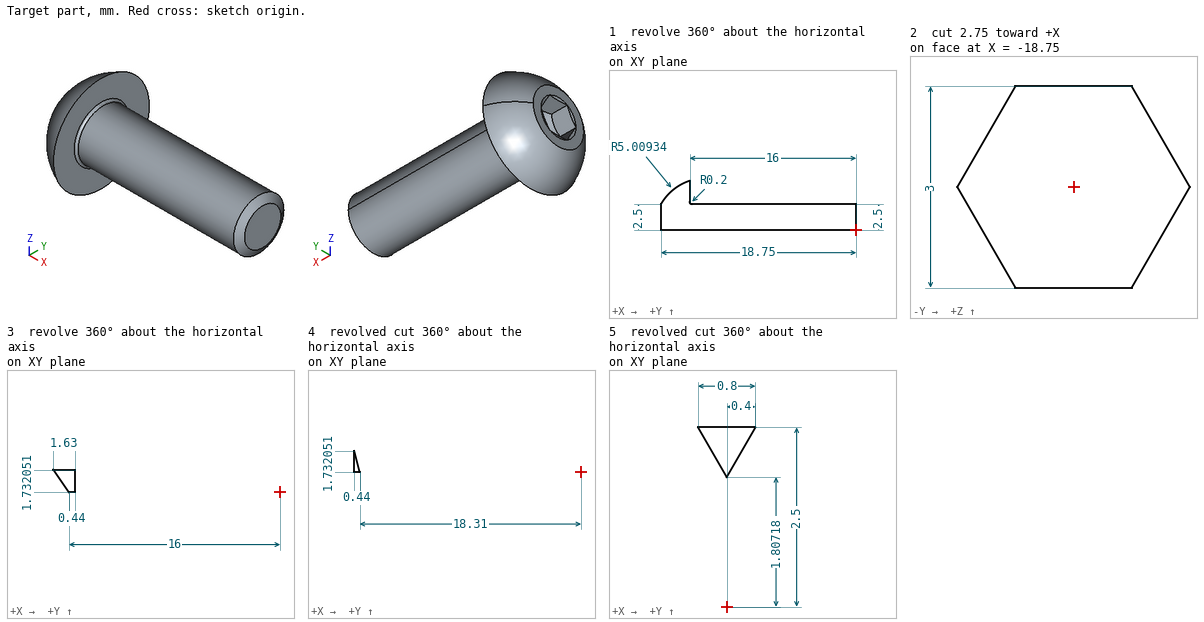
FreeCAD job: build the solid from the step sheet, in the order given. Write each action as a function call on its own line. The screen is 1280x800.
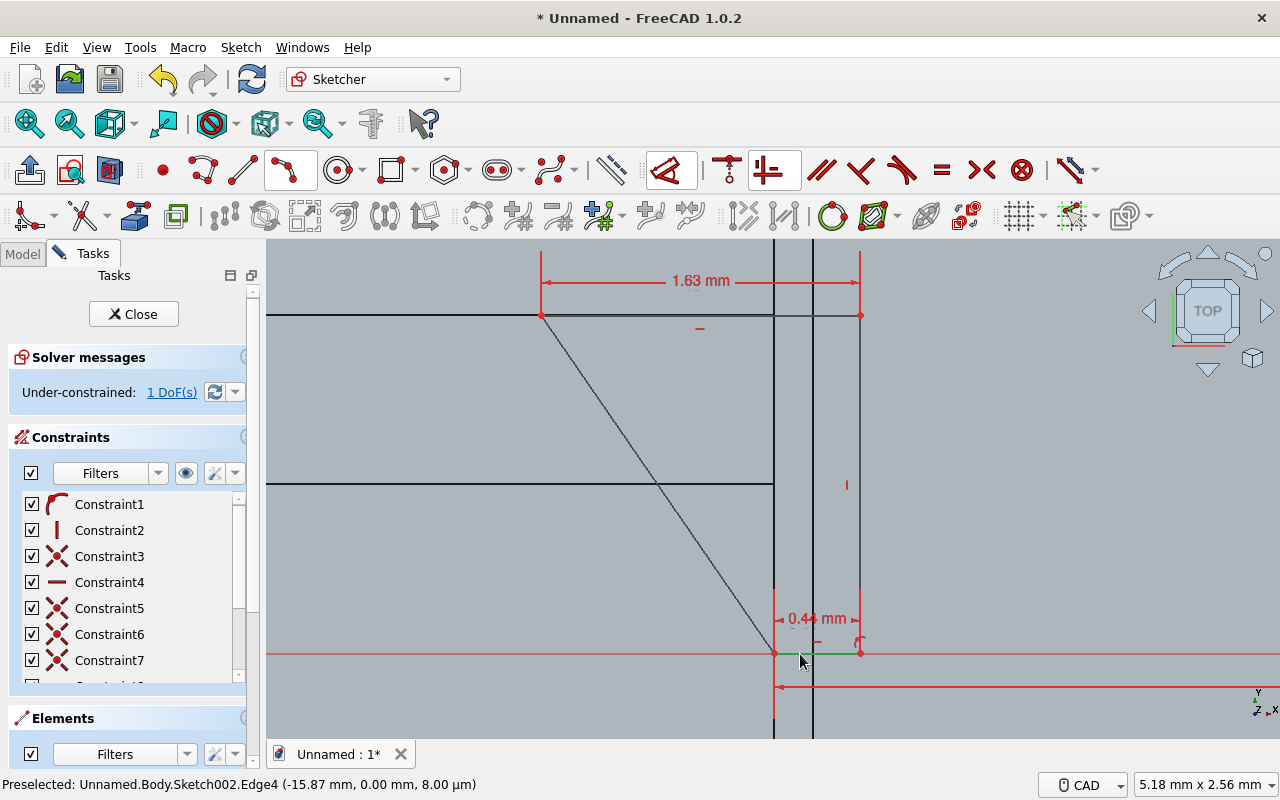
click(860, 552)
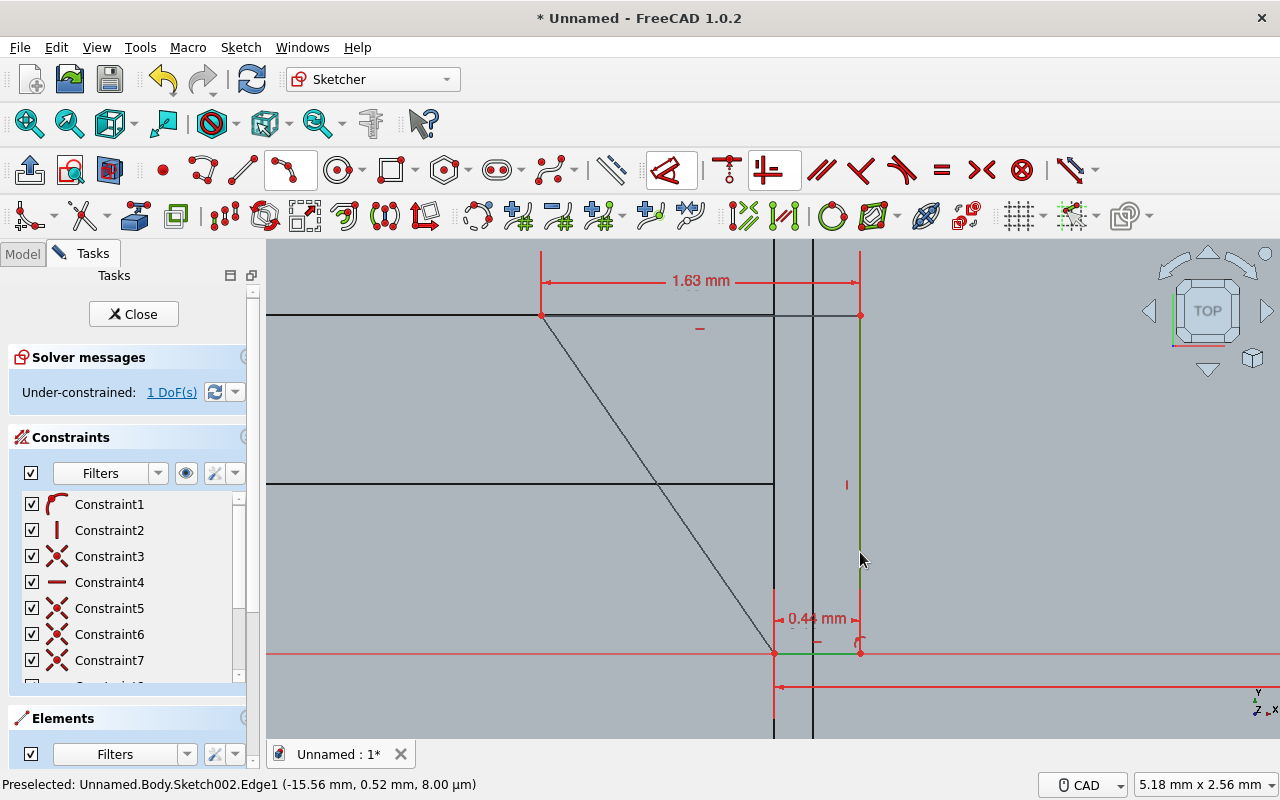
click(692, 170)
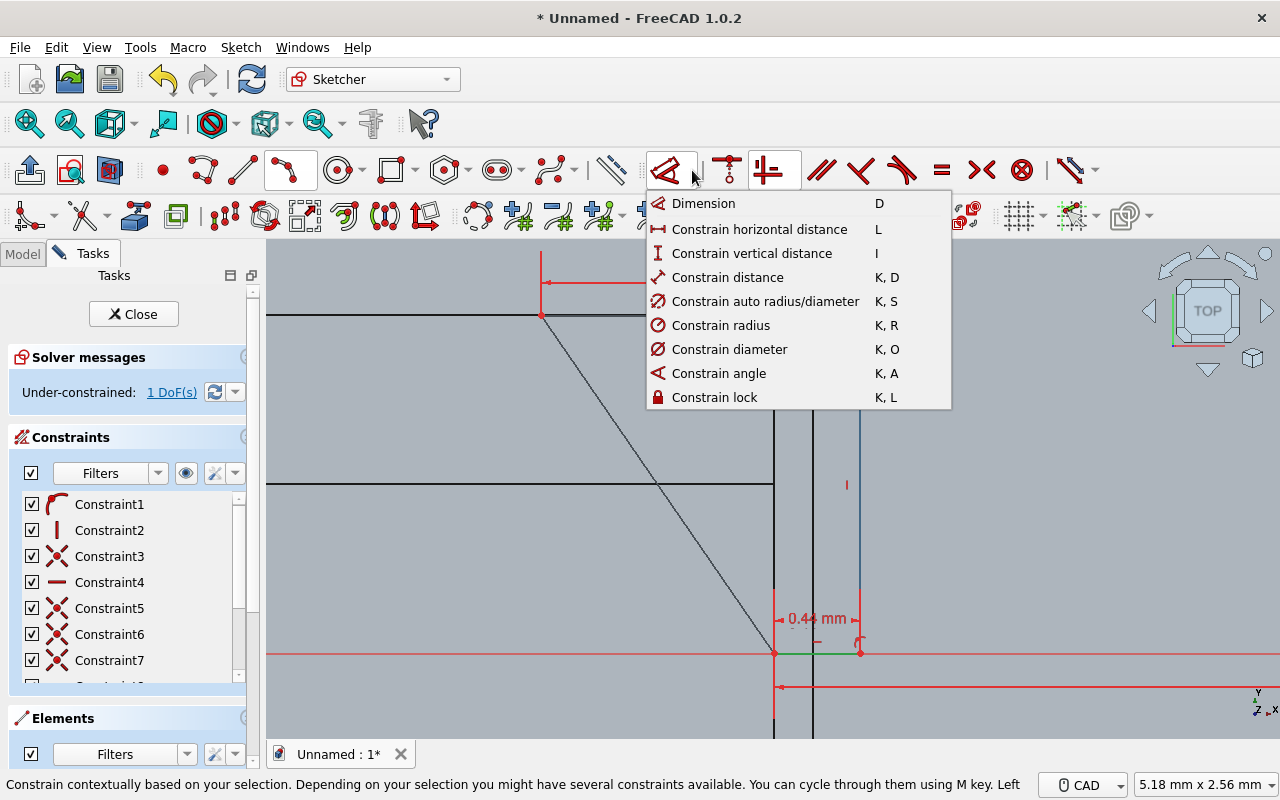
click(799, 253)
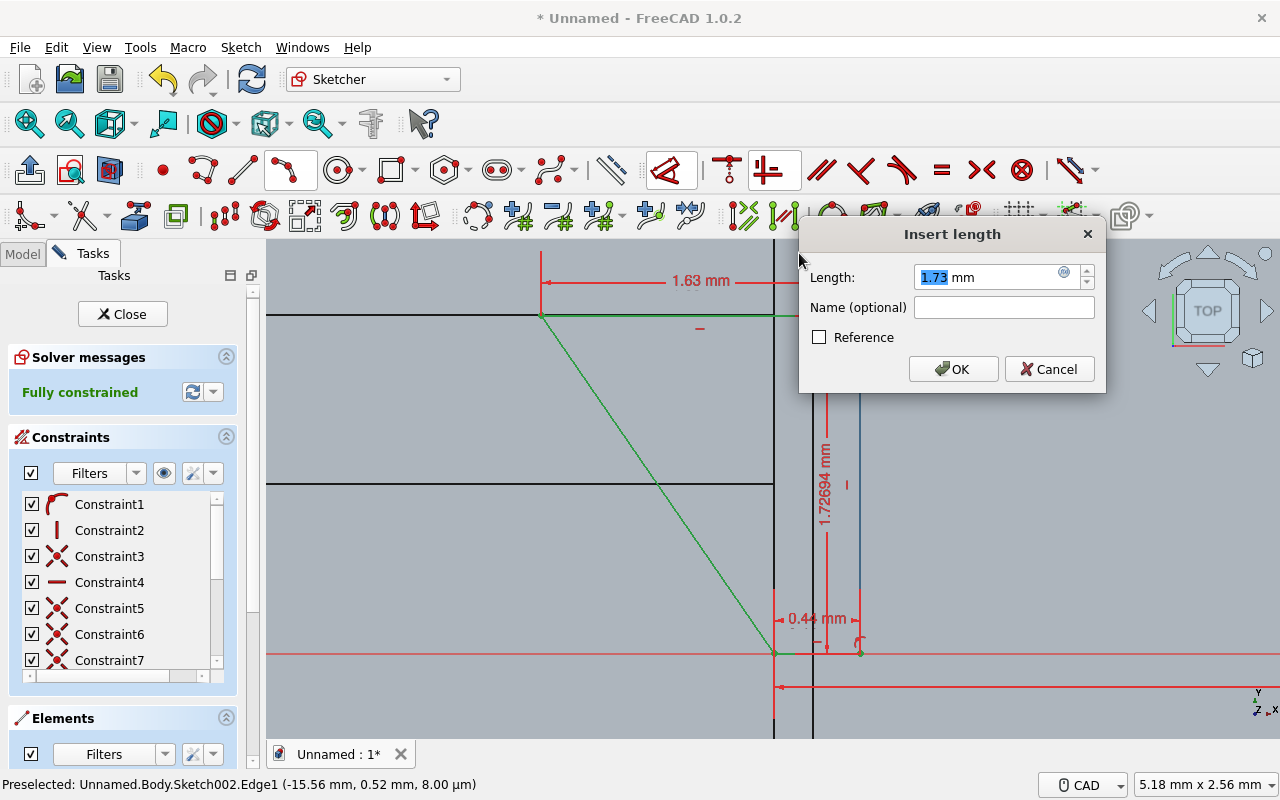
text(1.732051)
key(Return)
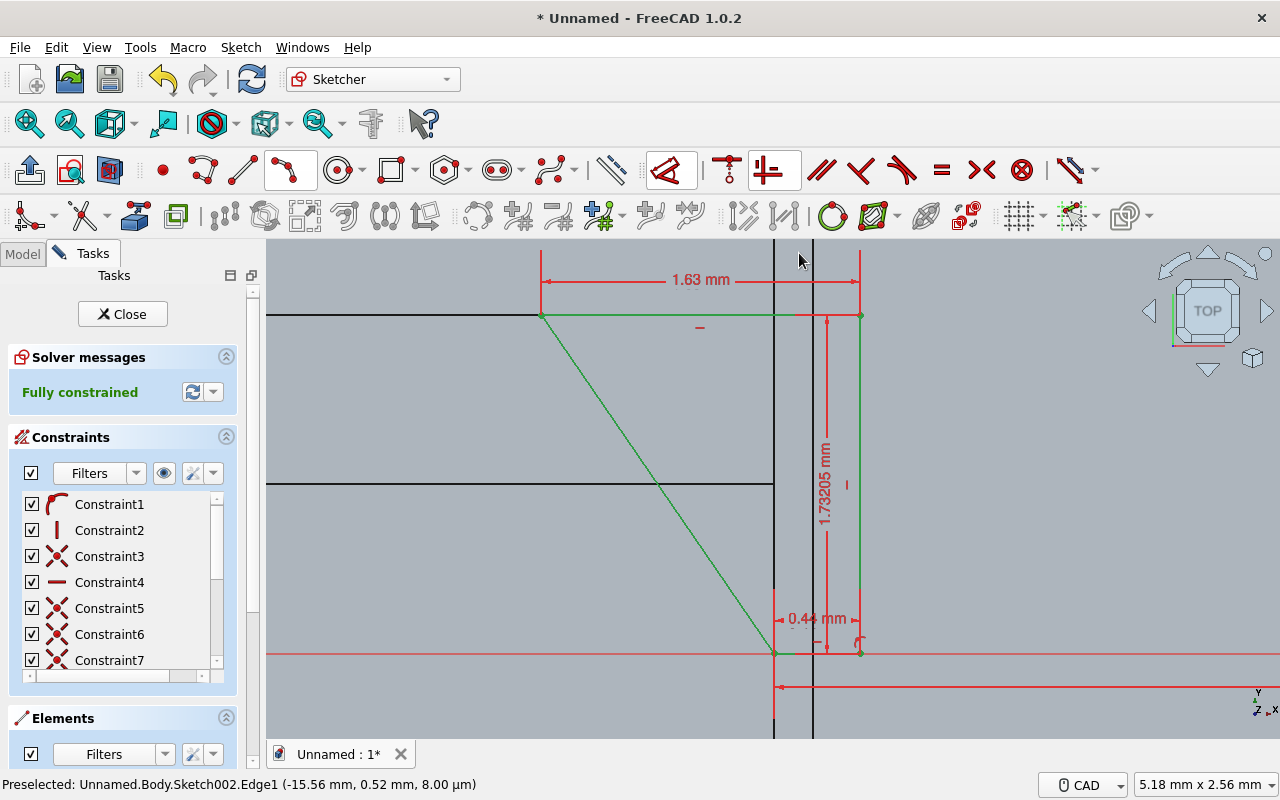
click(123, 314)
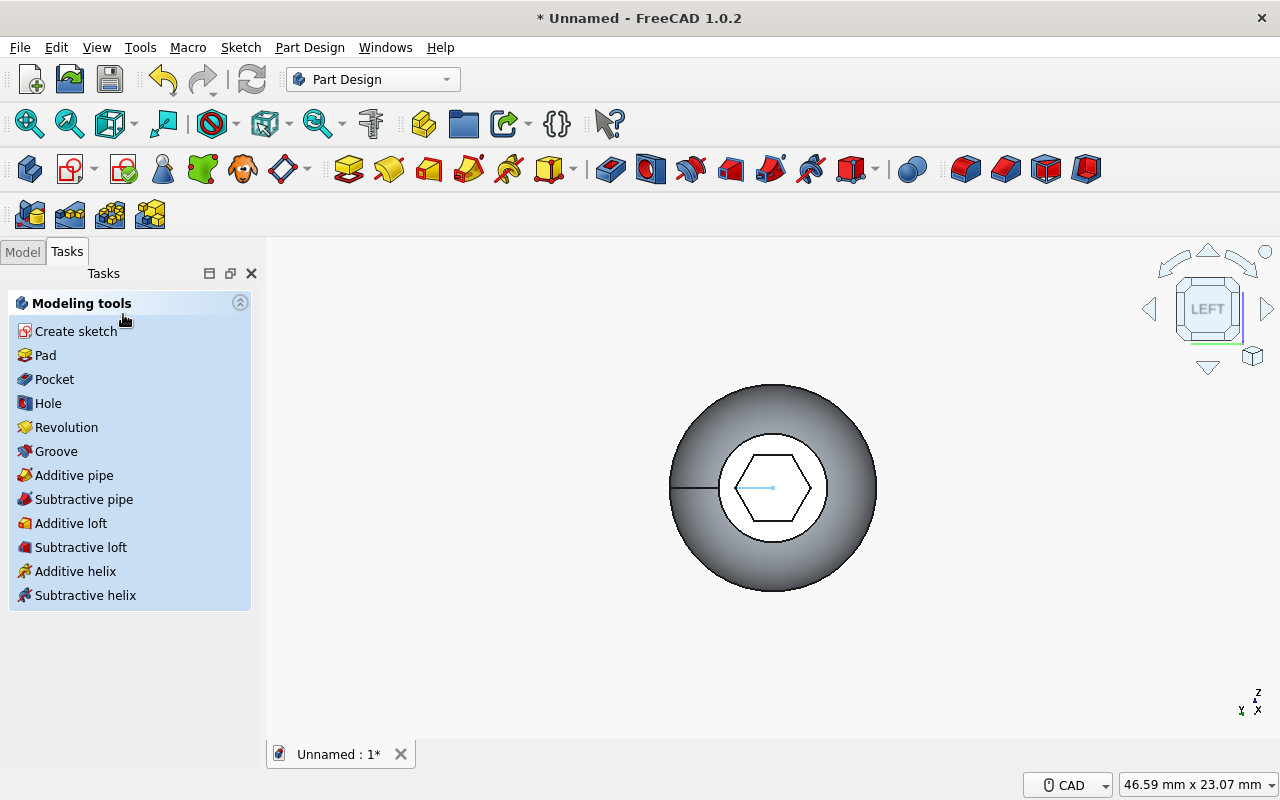
click(390, 170)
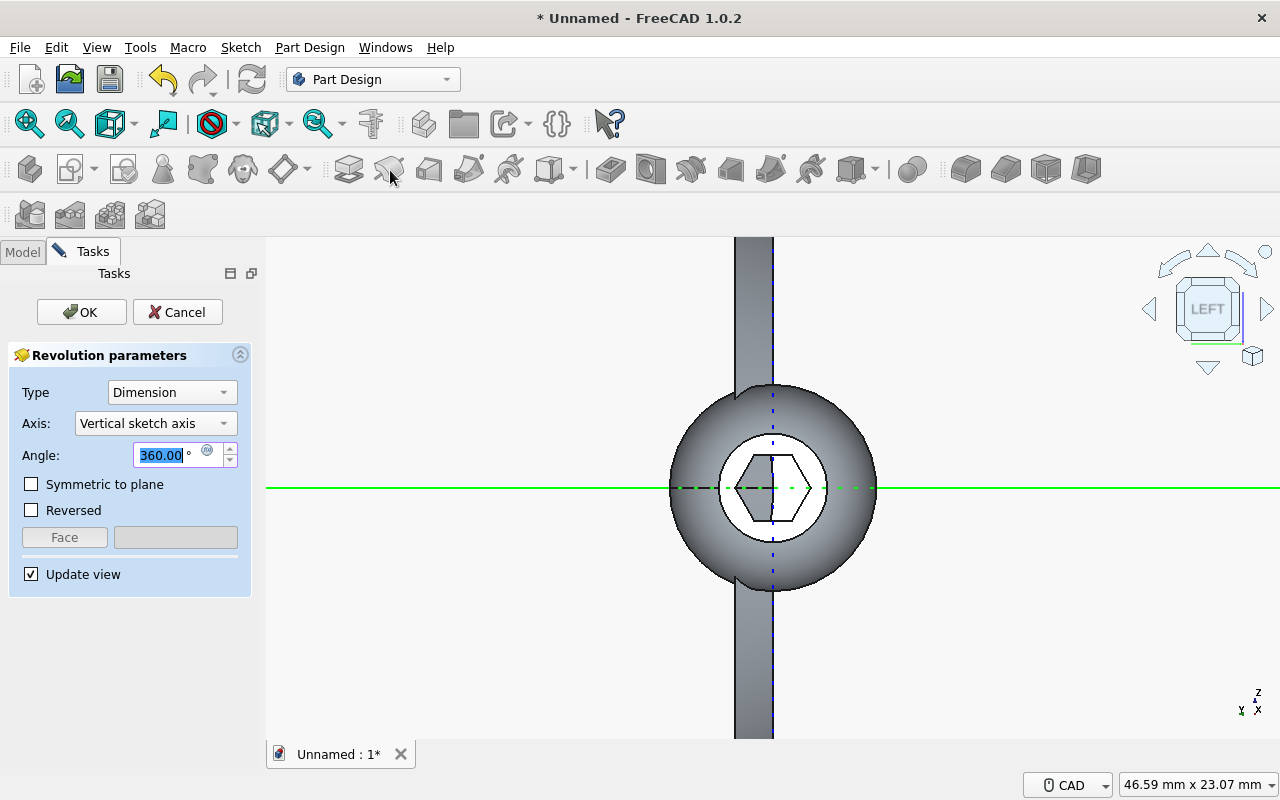
click(156, 424)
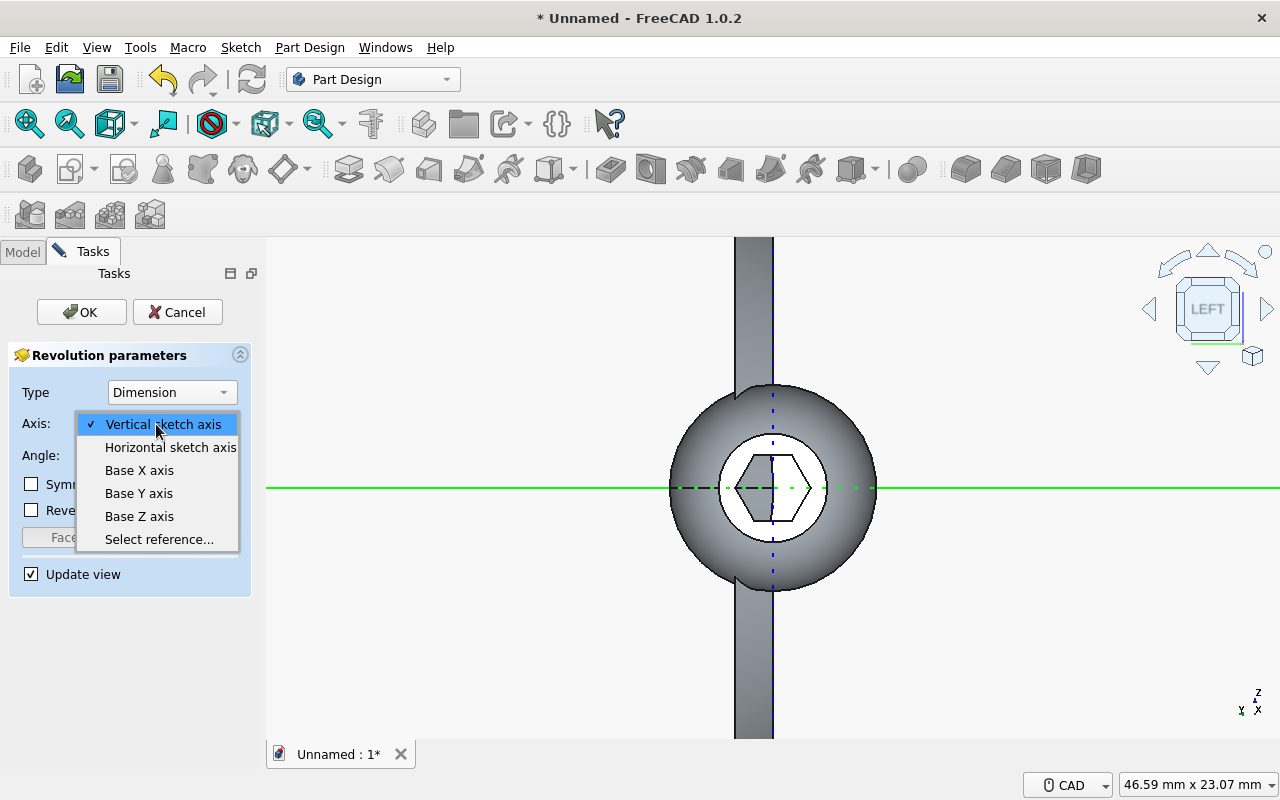
click(156, 448)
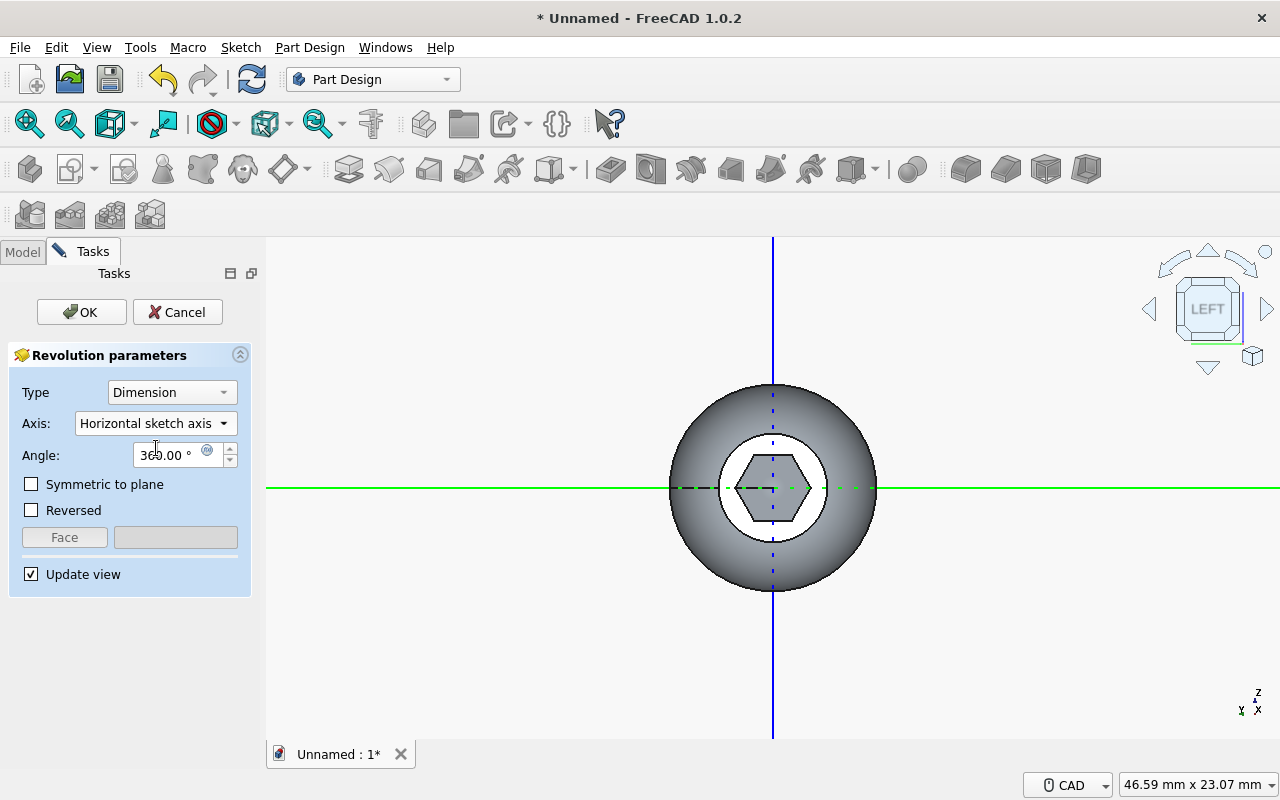
click(82, 312)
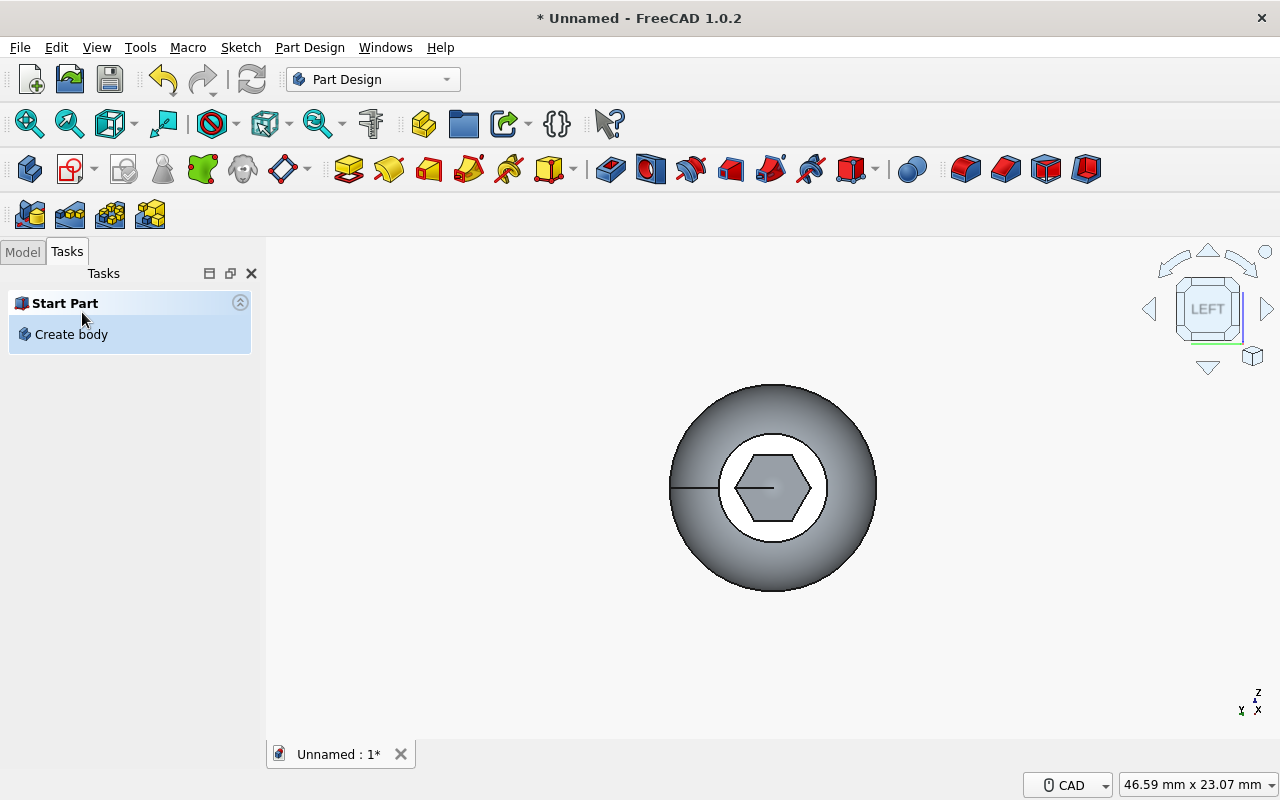
click(30, 124)